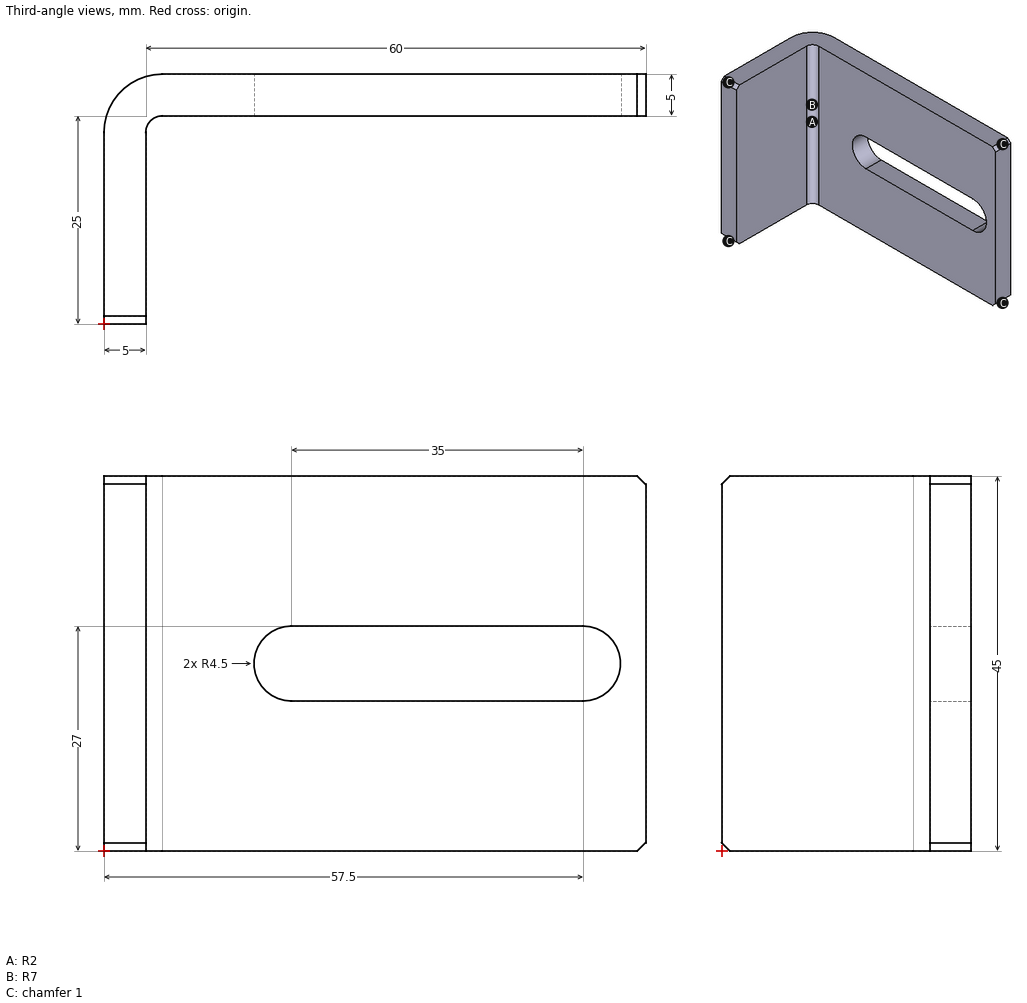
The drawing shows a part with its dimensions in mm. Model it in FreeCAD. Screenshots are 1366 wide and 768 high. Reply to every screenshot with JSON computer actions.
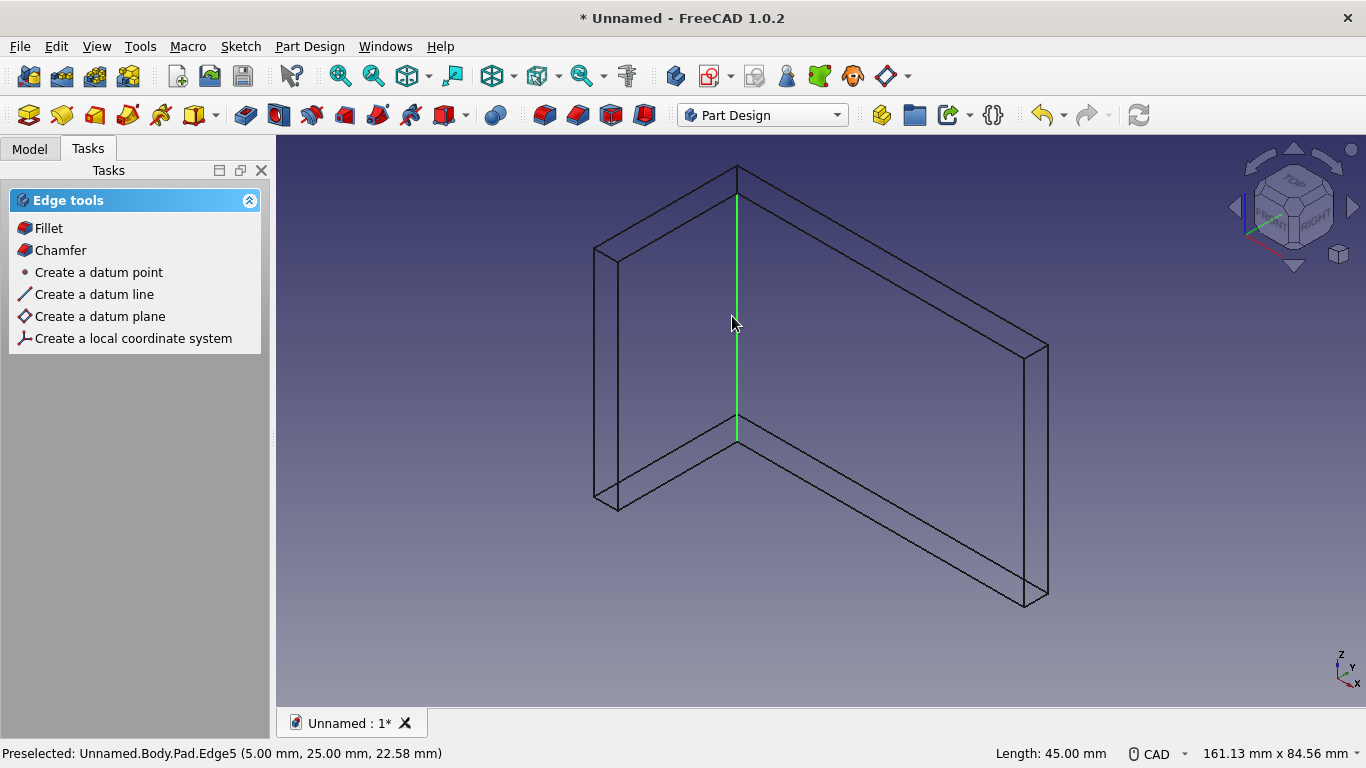
{"action": "key", "text": "v 1"}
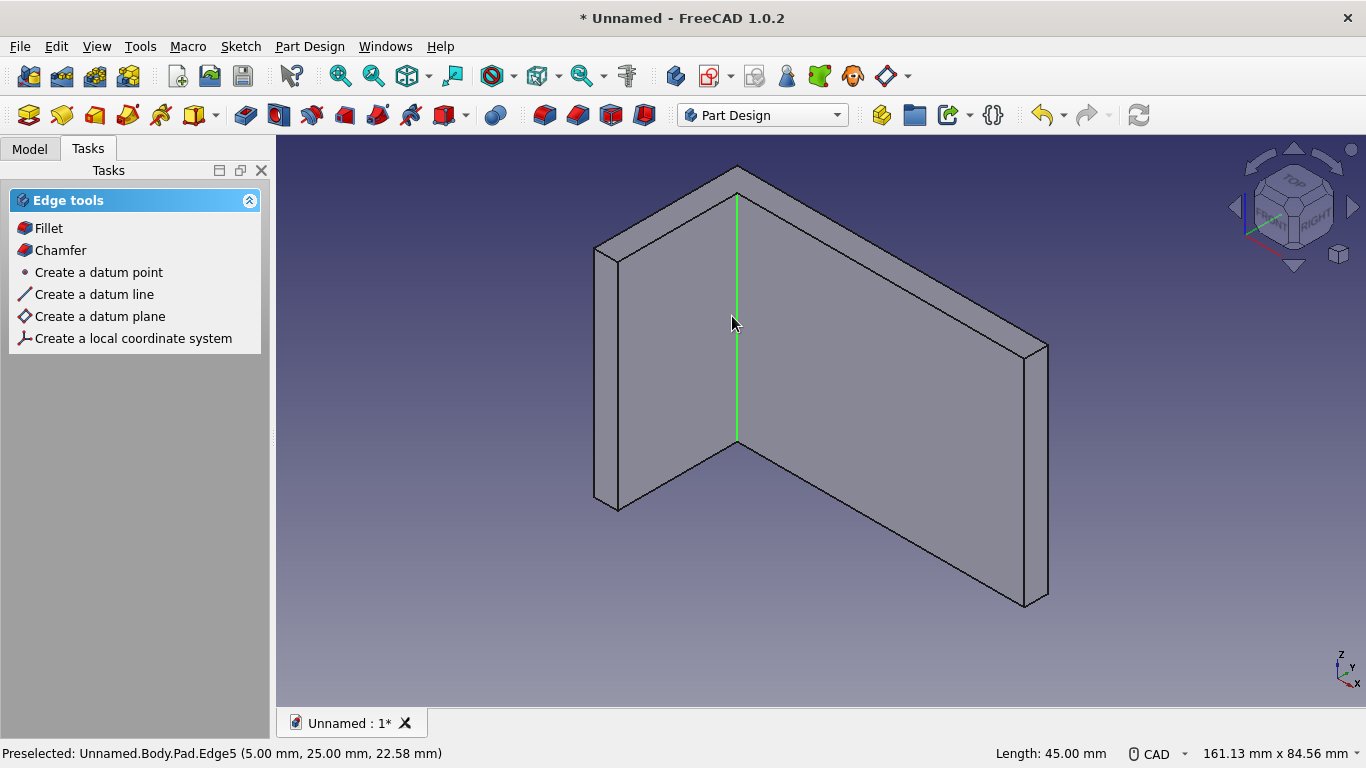
{"action": "left_click", "coordinate": [545, 116]}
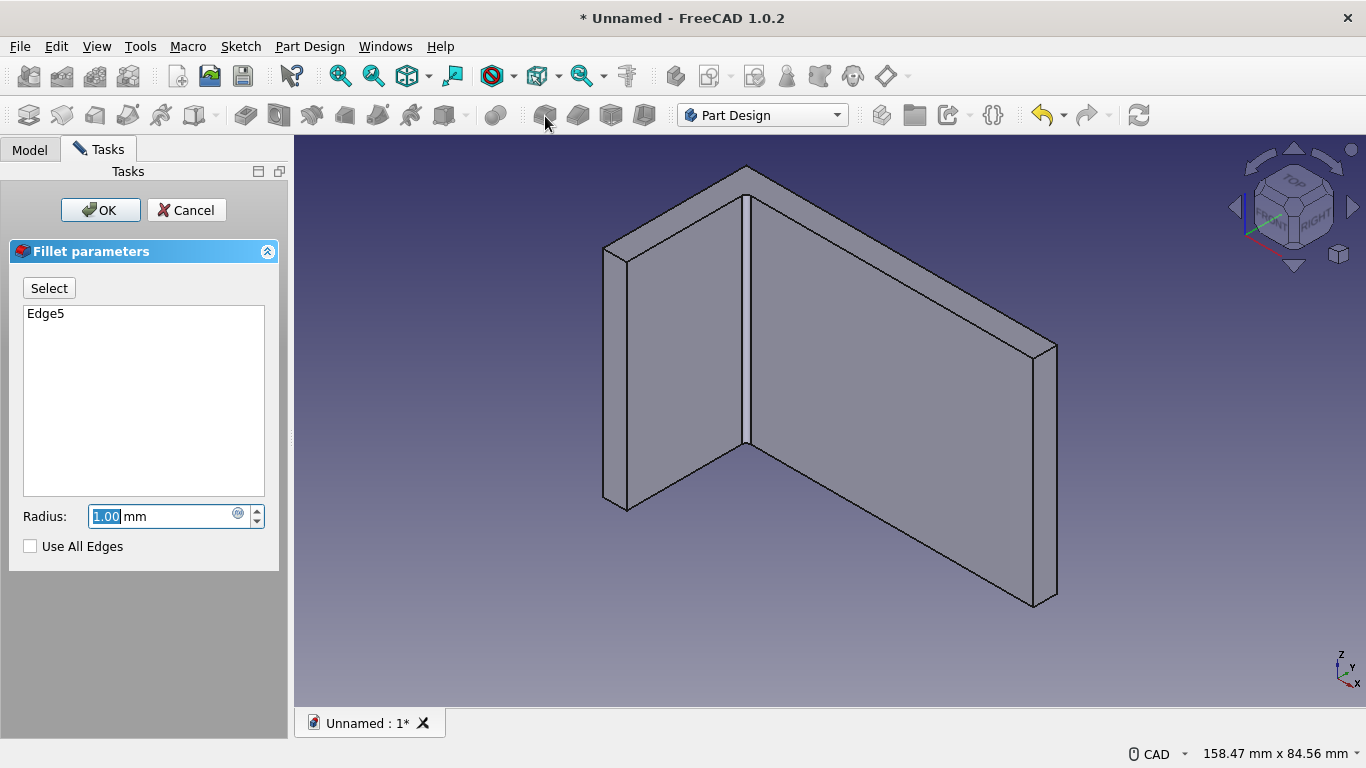
{"action": "type", "text": "2"}
{"action": "key", "text": "Tab"}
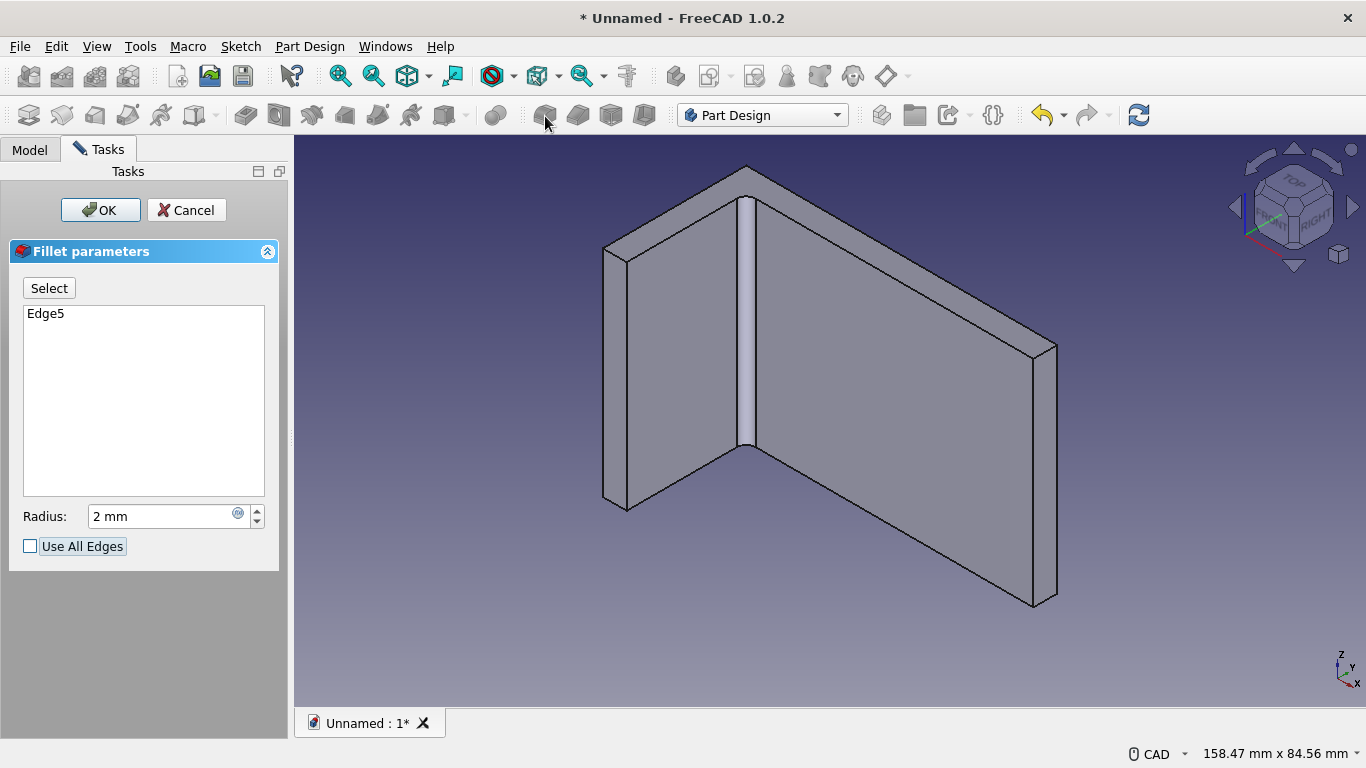
{"action": "left_click", "coordinate": [101, 210]}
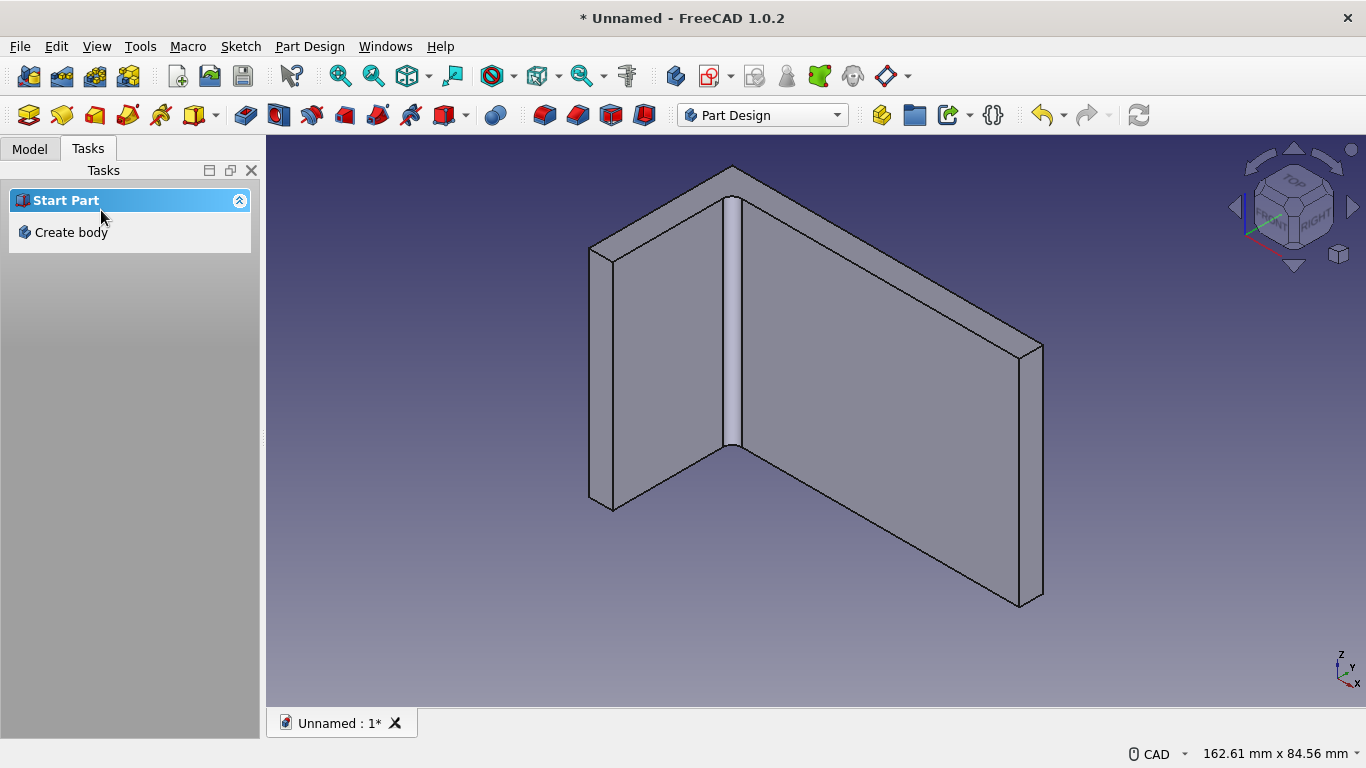
{"action": "key", "text": "2"}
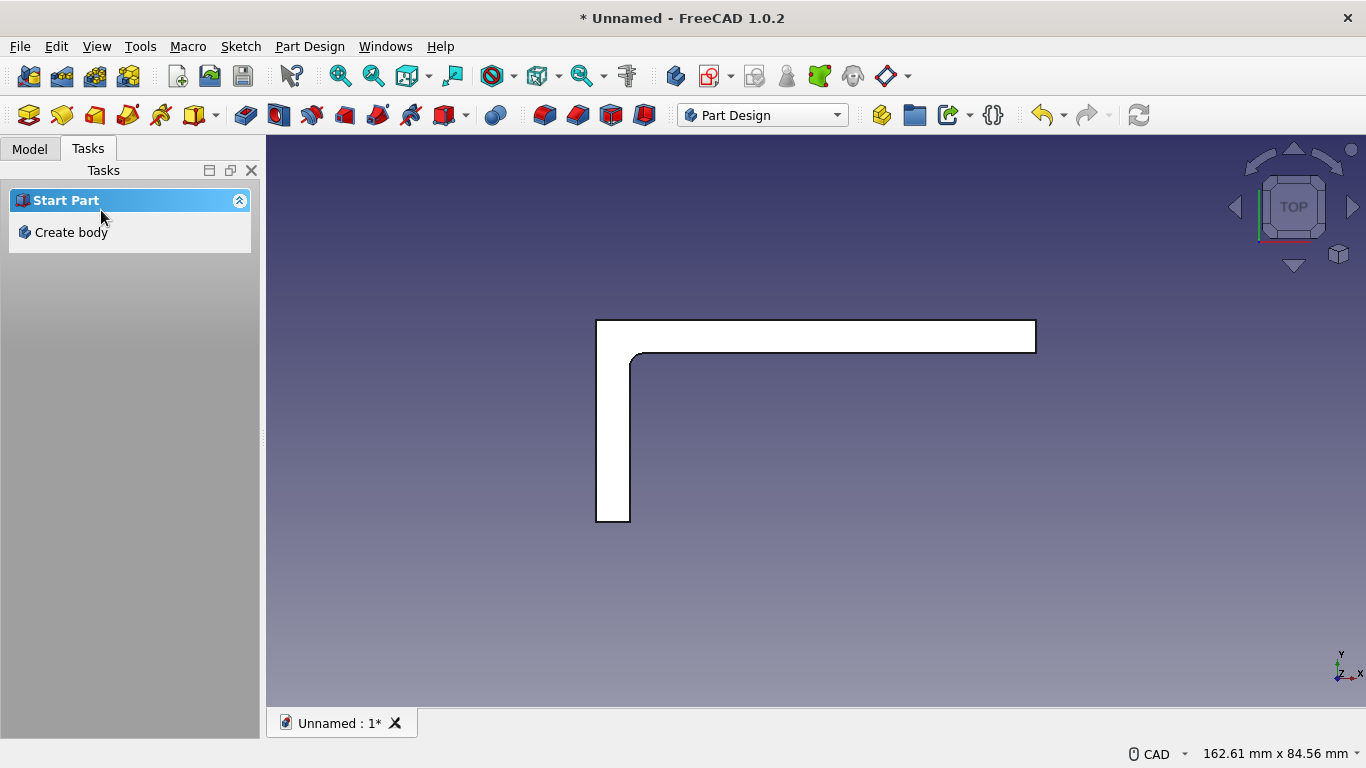
{"action": "left_click", "coordinate": [341, 76]}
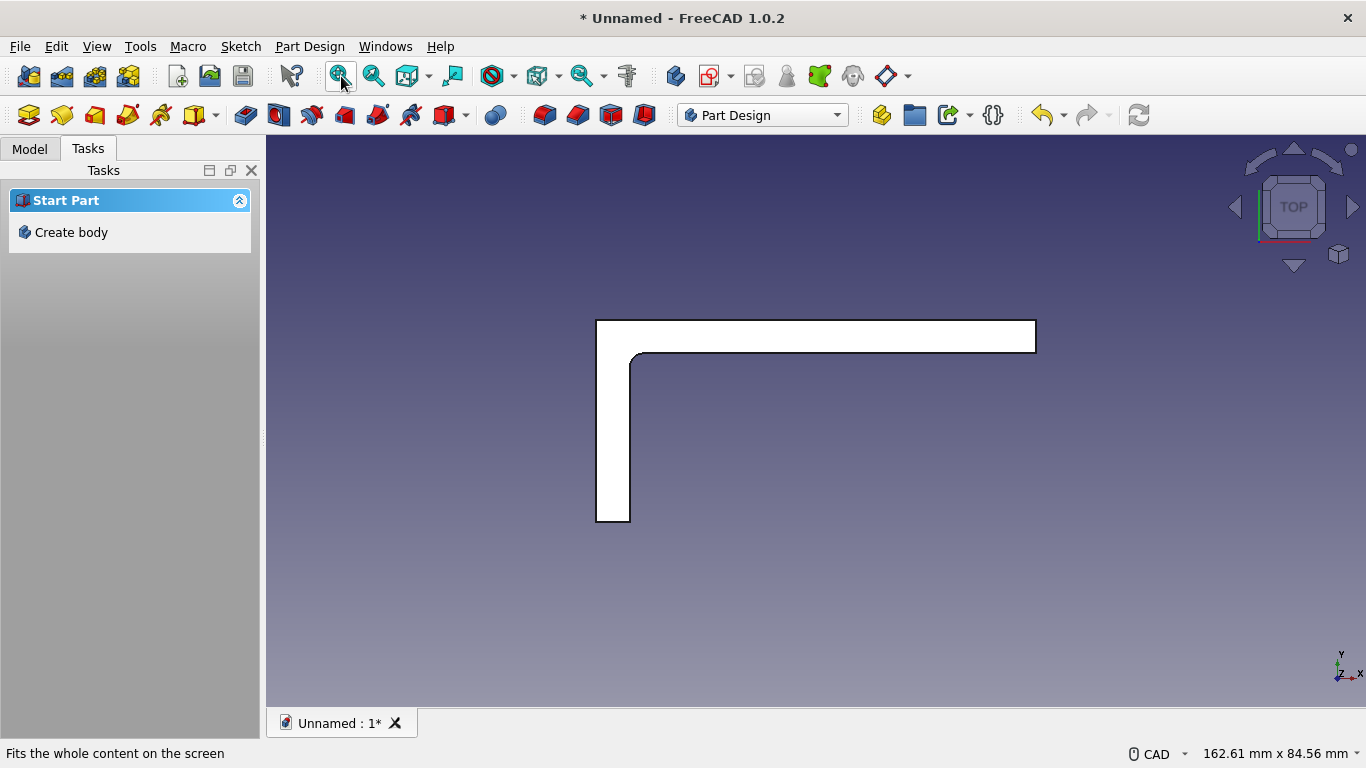
{"action": "key", "text": "0"}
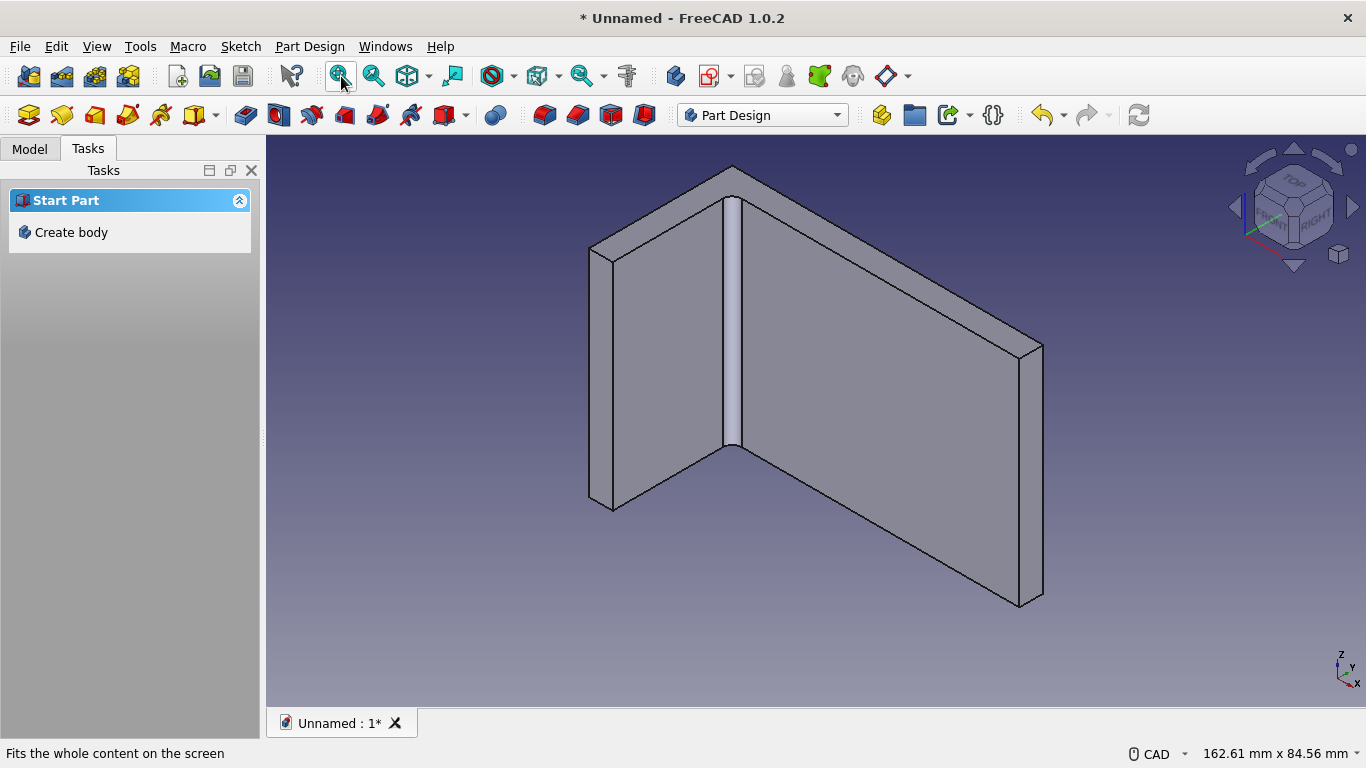
{"action": "key", "text": "1"}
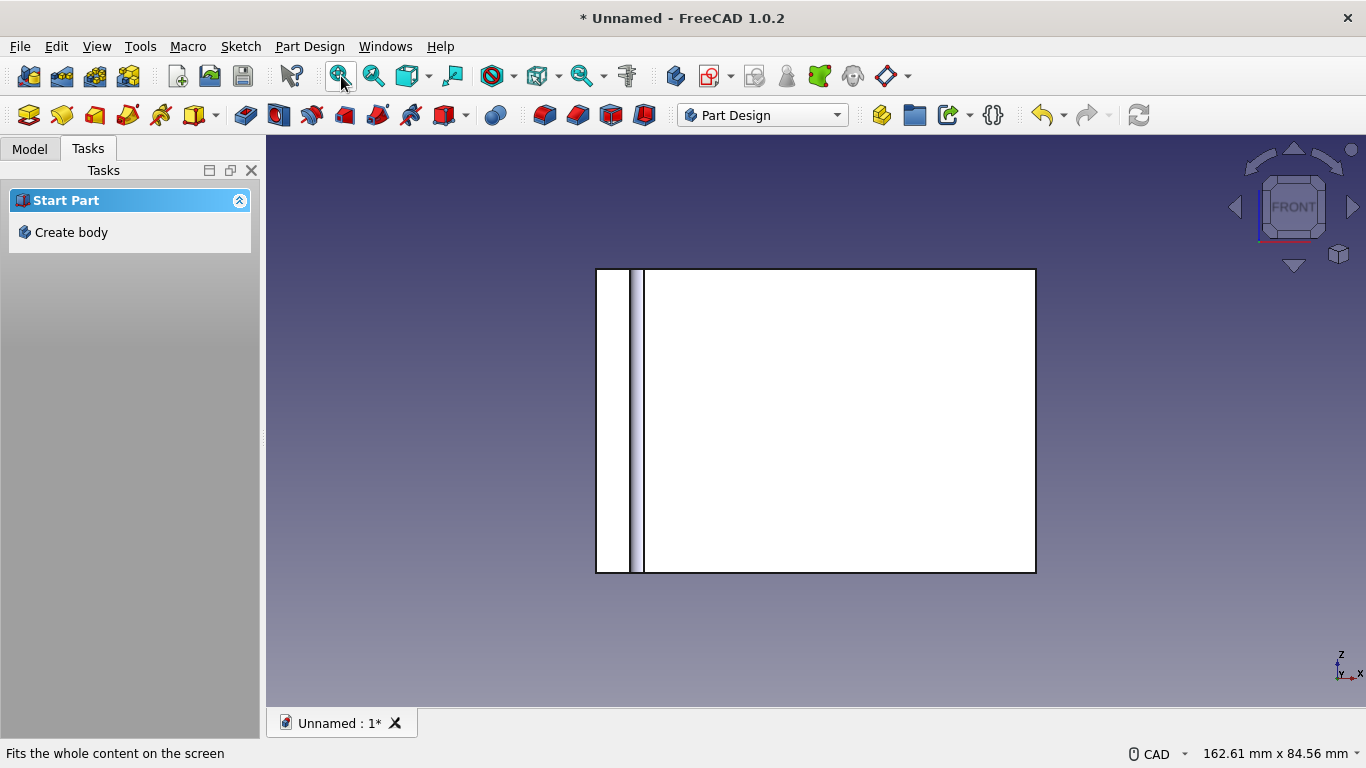
{"action": "key", "text": "3"}